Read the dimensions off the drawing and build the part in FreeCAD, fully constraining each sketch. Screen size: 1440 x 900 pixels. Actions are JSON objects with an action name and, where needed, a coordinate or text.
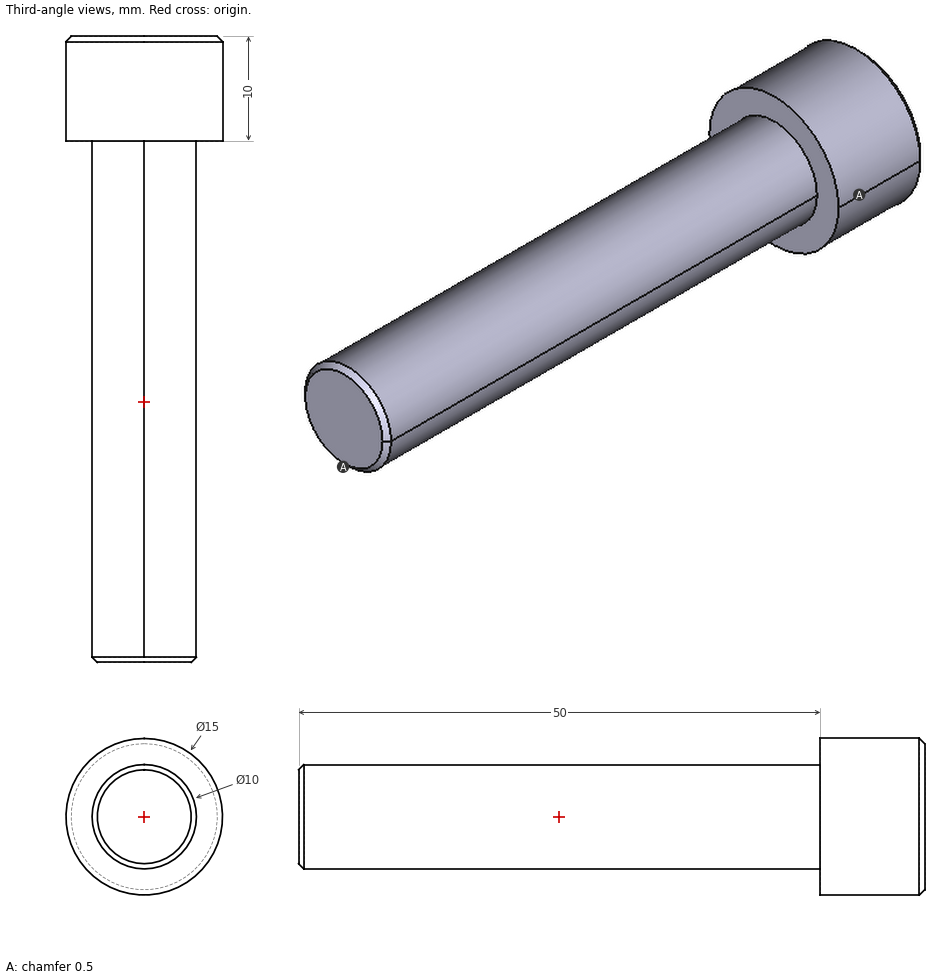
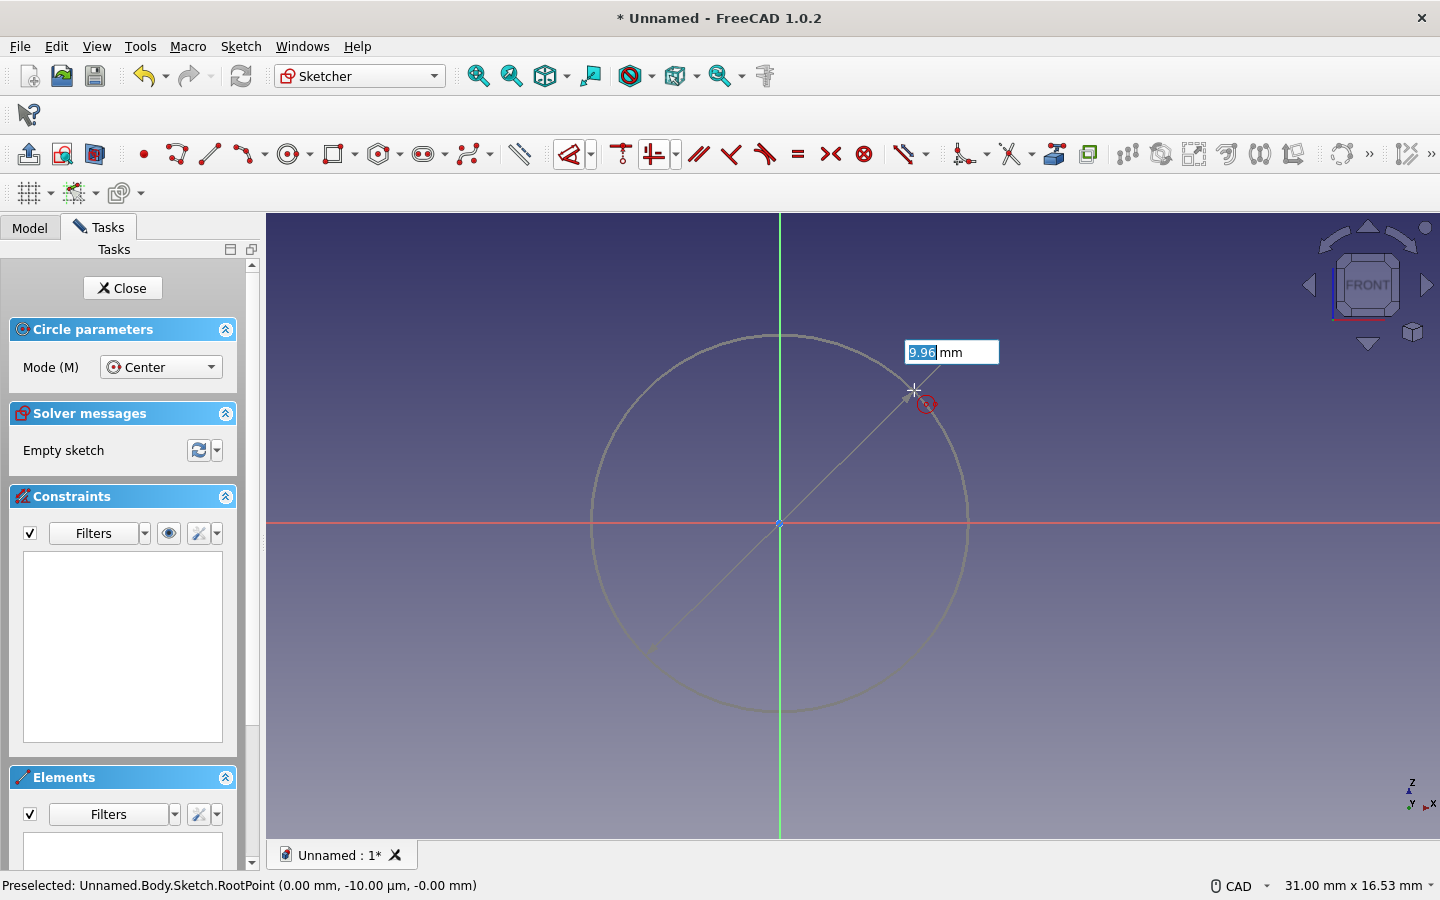
{"action": "type", "text": "10"}
{"action": "key", "text": "Return"}
{"action": "key", "text": "Escape"}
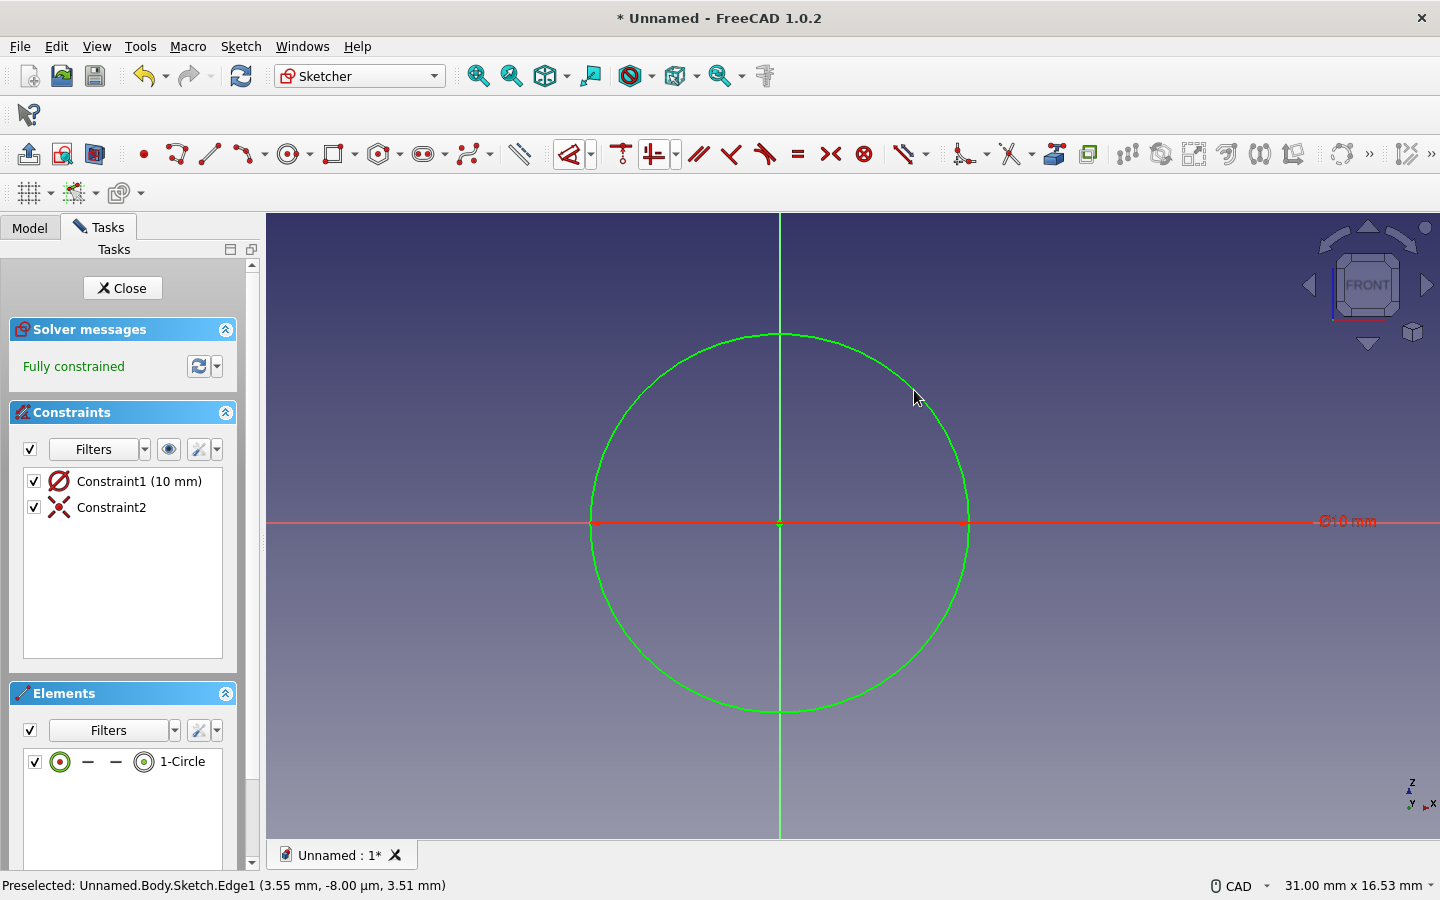
{"action": "left_click", "coordinate": [123, 288]}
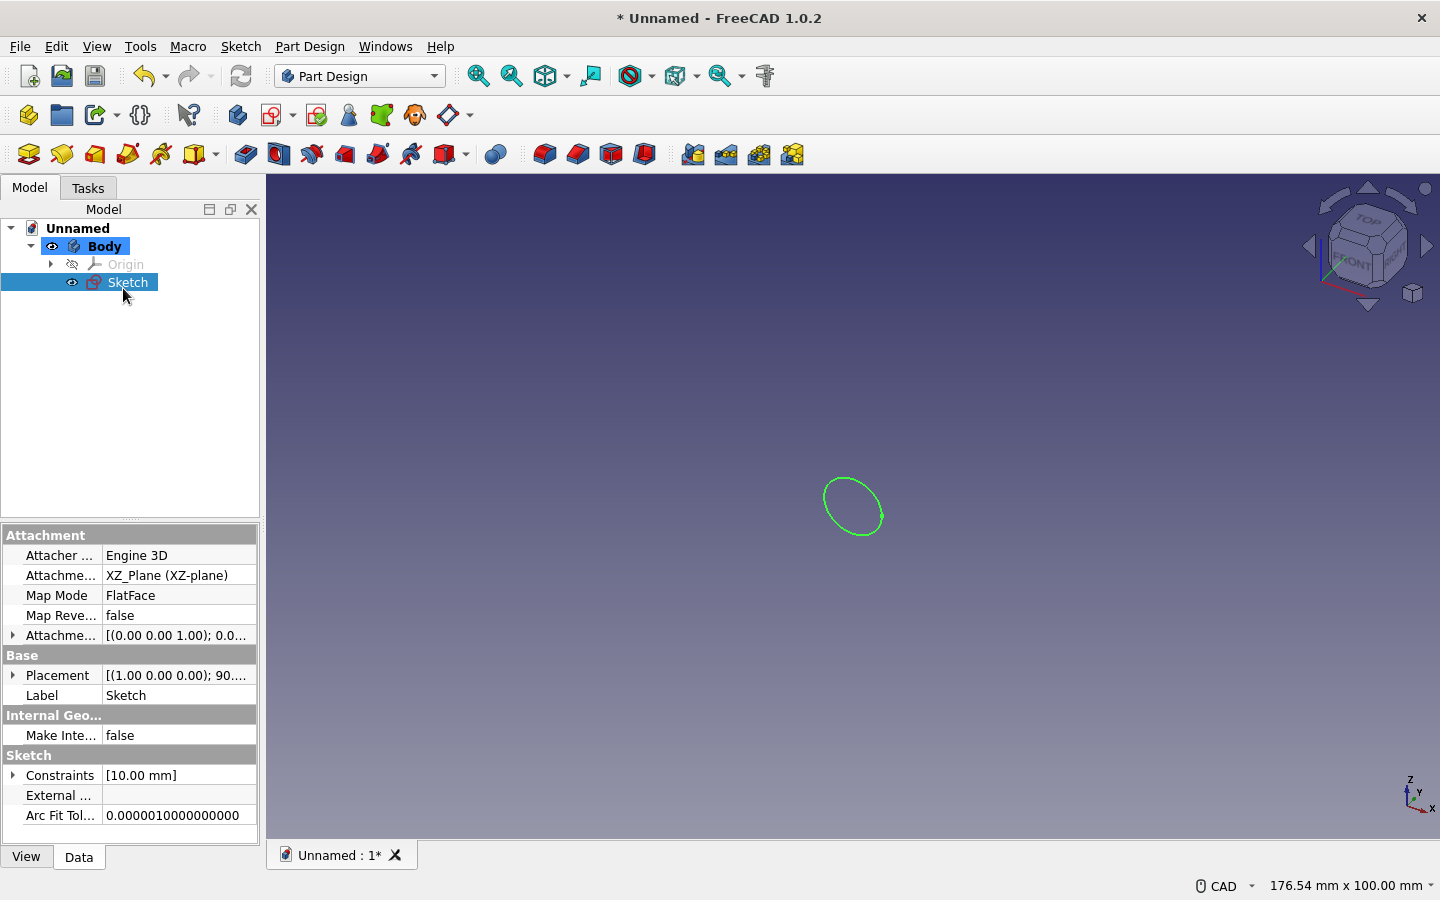
{"action": "left_click", "coordinate": [29, 154]}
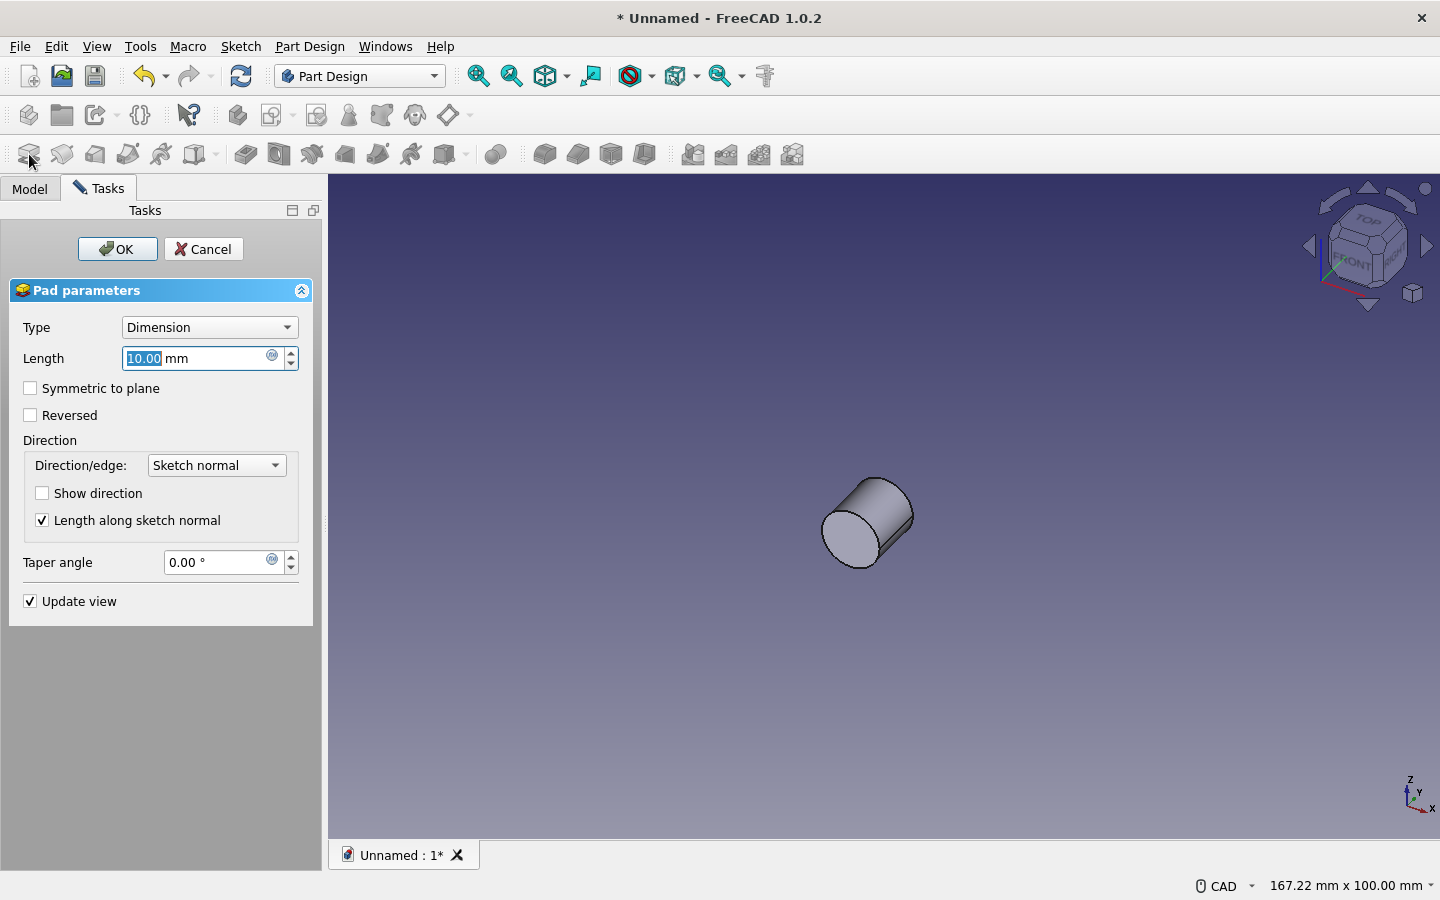
{"action": "type", "text": "50"}
{"action": "key", "text": "Tab"}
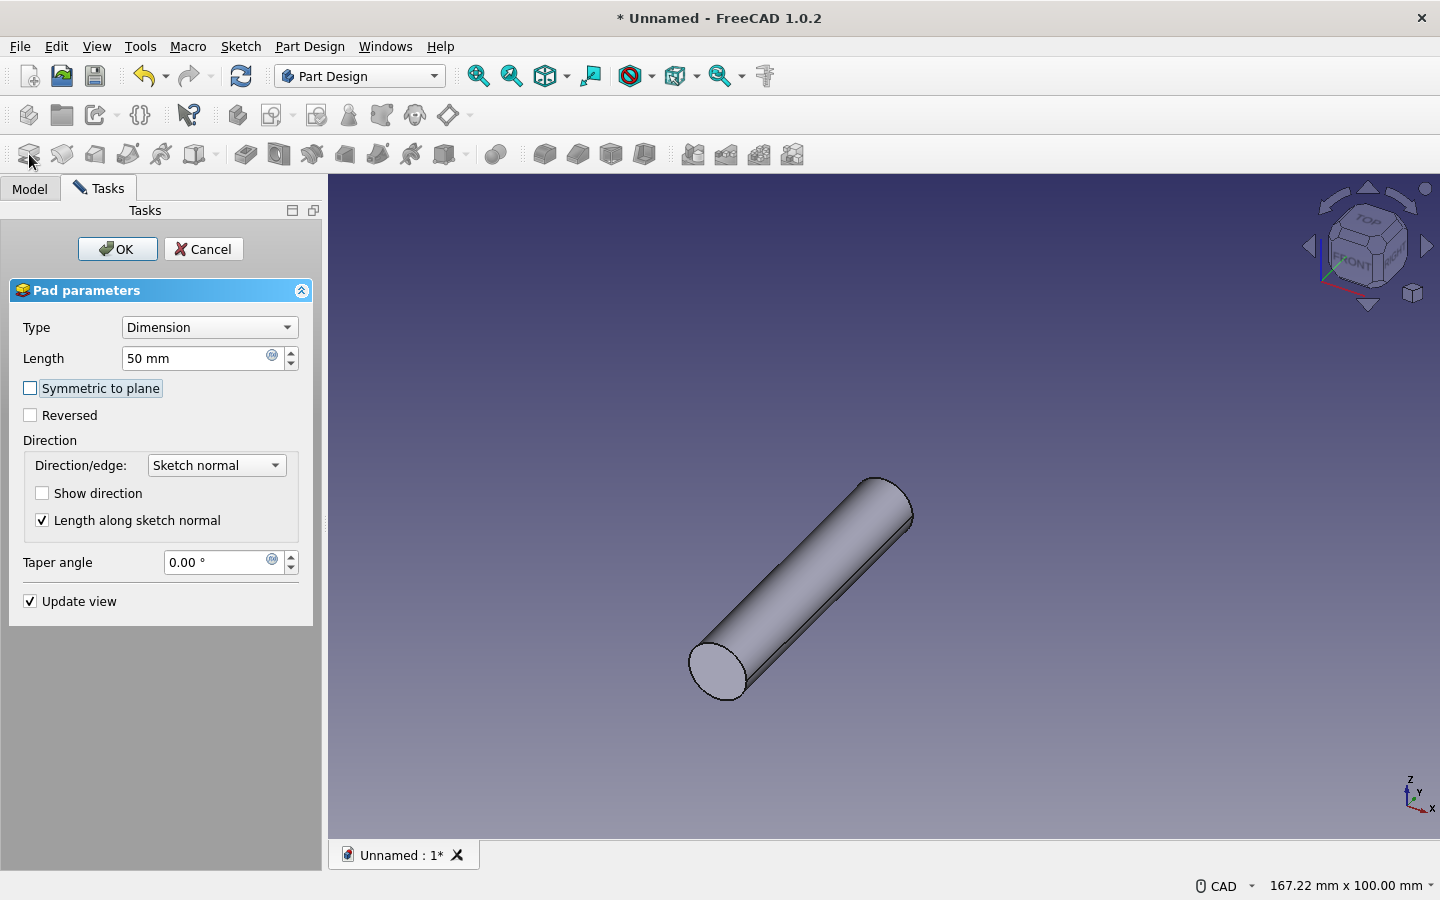
{"action": "left_click", "coordinate": [31, 388]}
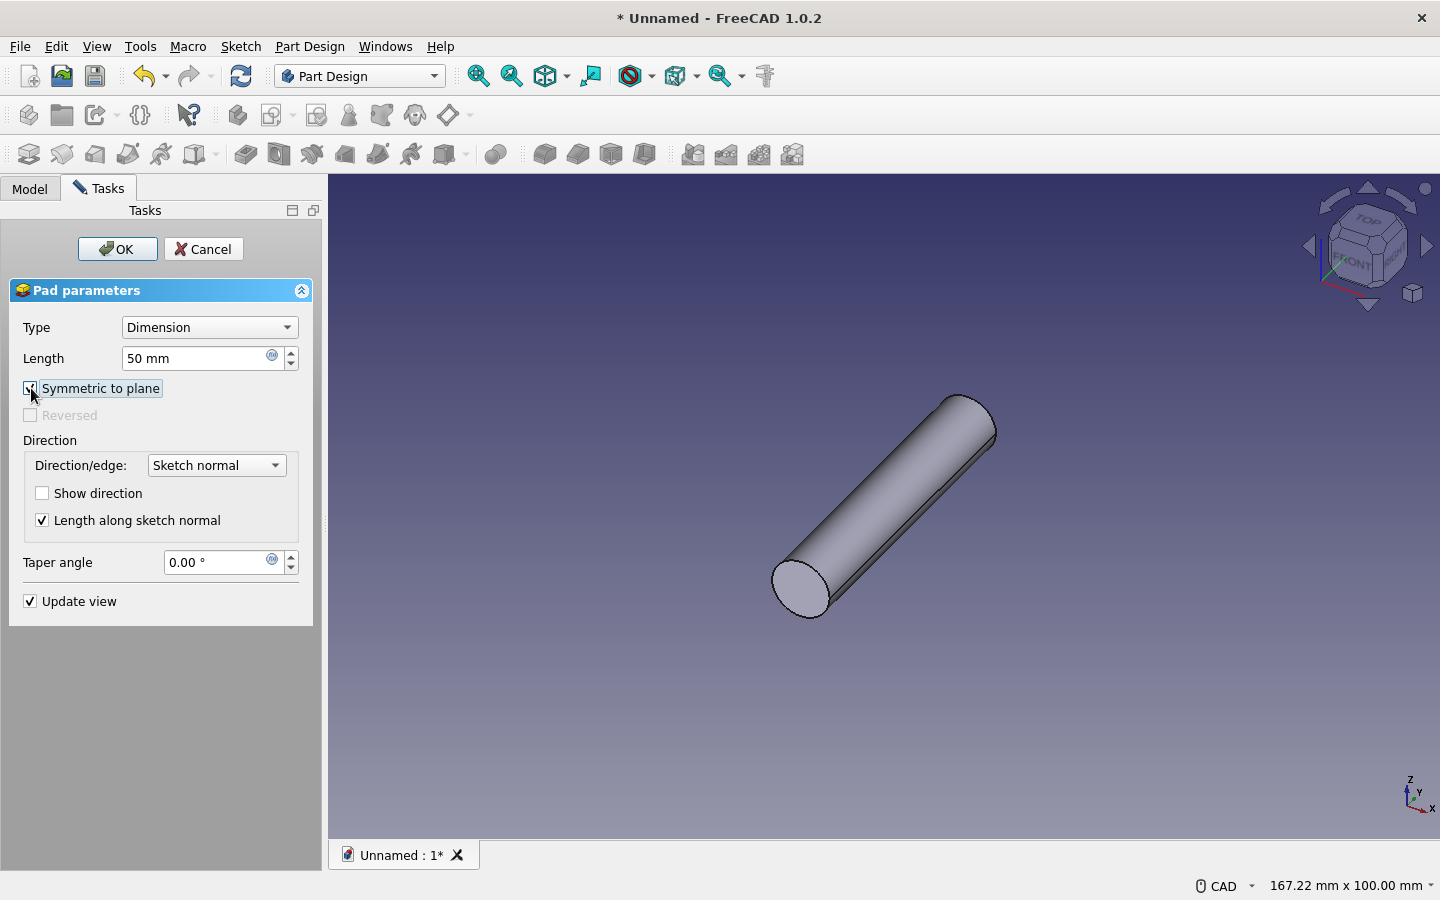
{"action": "left_click", "coordinate": [118, 249]}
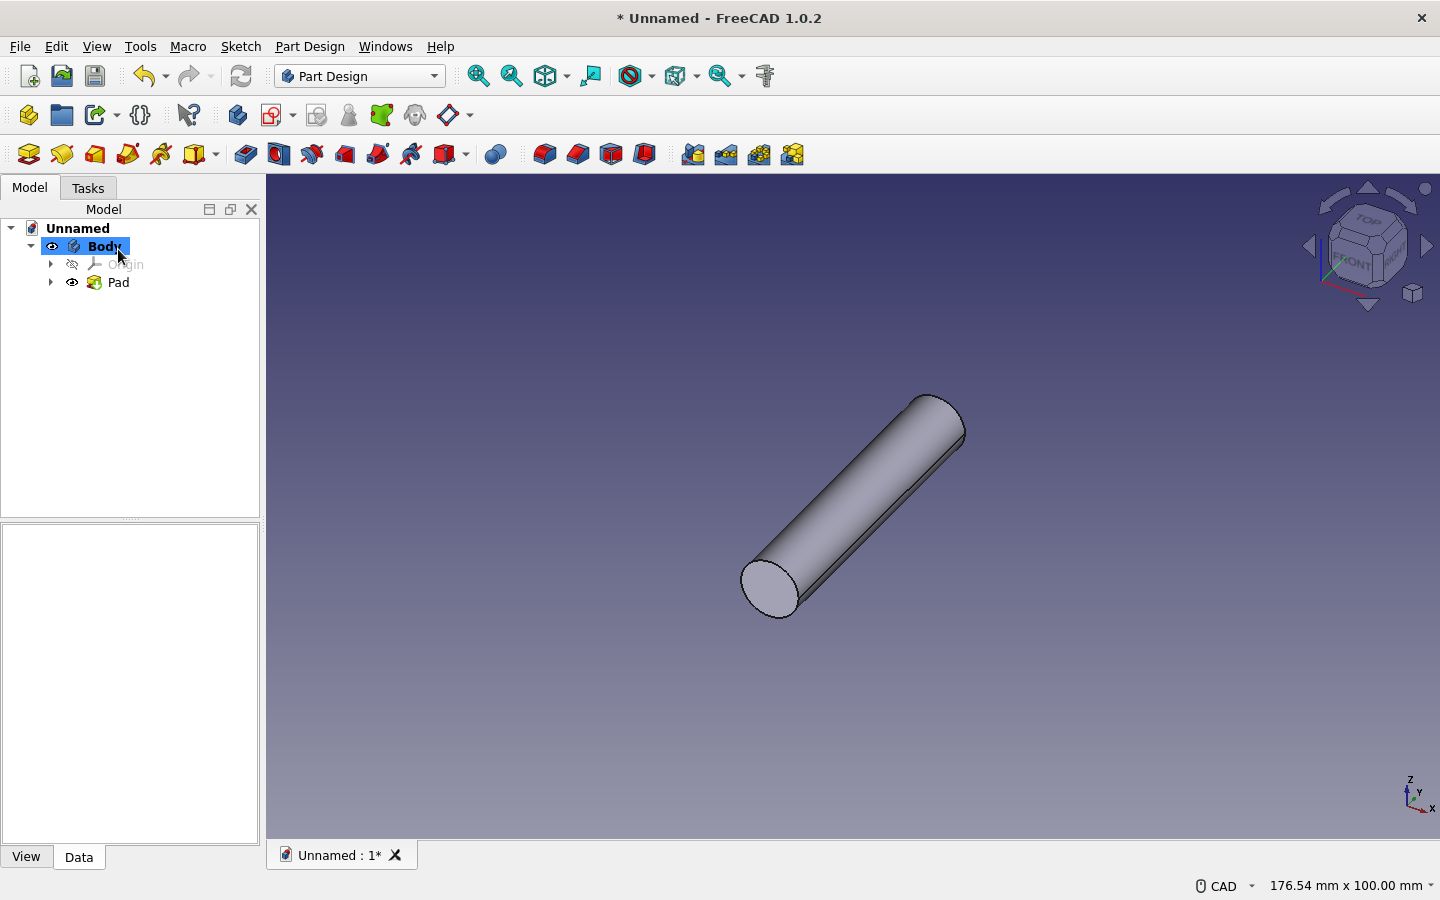
{"action": "left_click", "coordinate": [479, 76]}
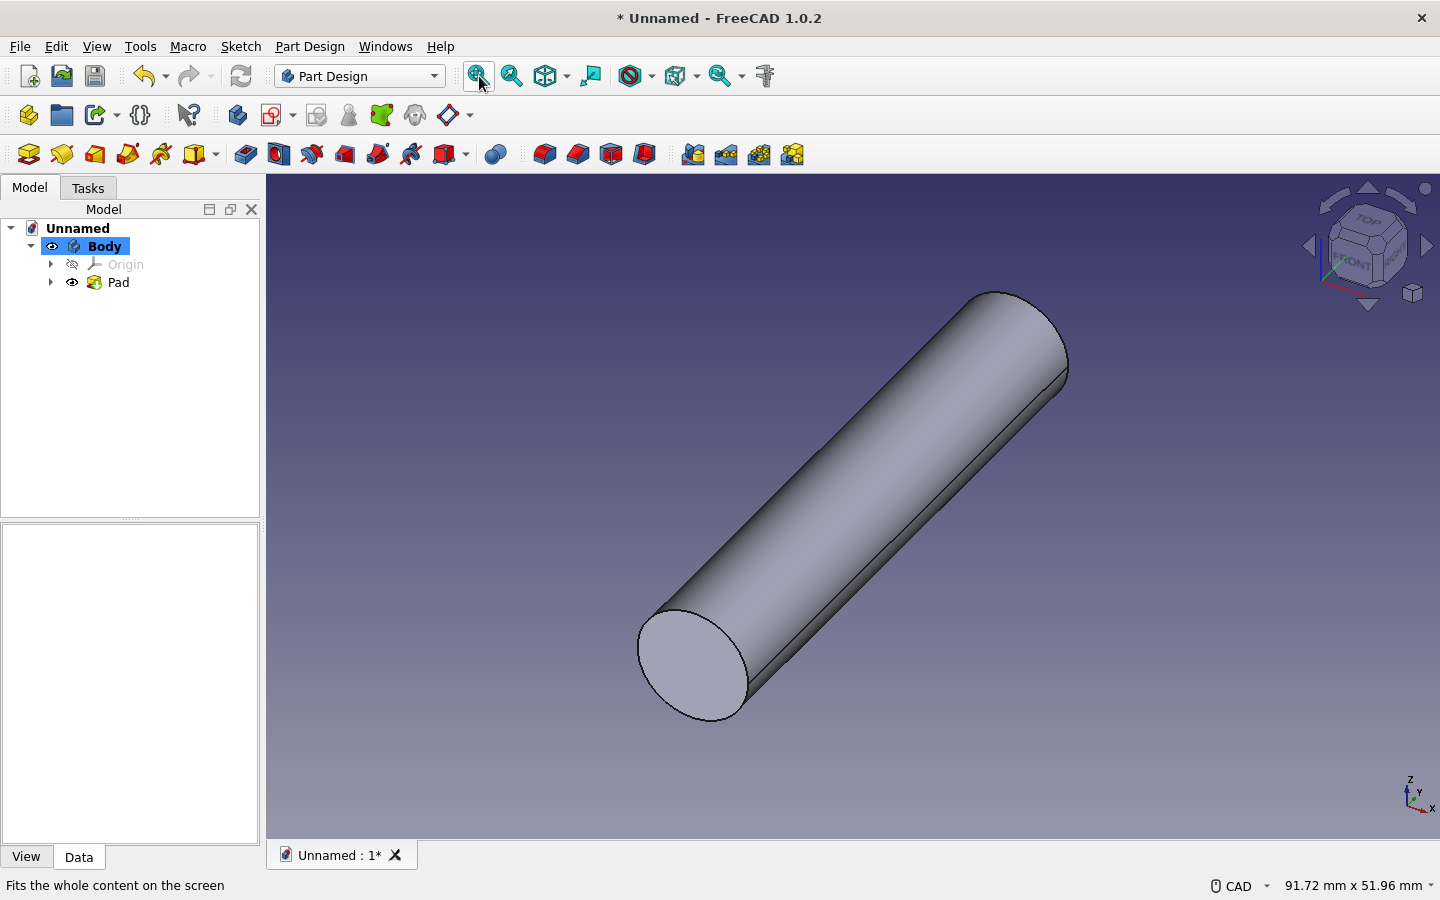
{"action": "key", "text": "4"}